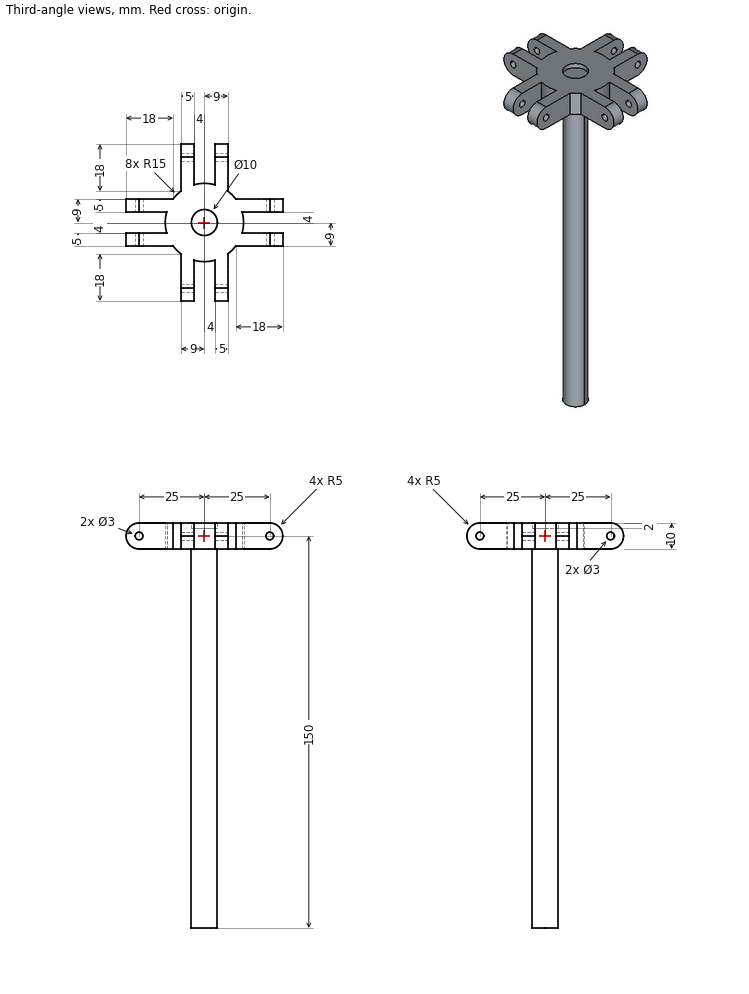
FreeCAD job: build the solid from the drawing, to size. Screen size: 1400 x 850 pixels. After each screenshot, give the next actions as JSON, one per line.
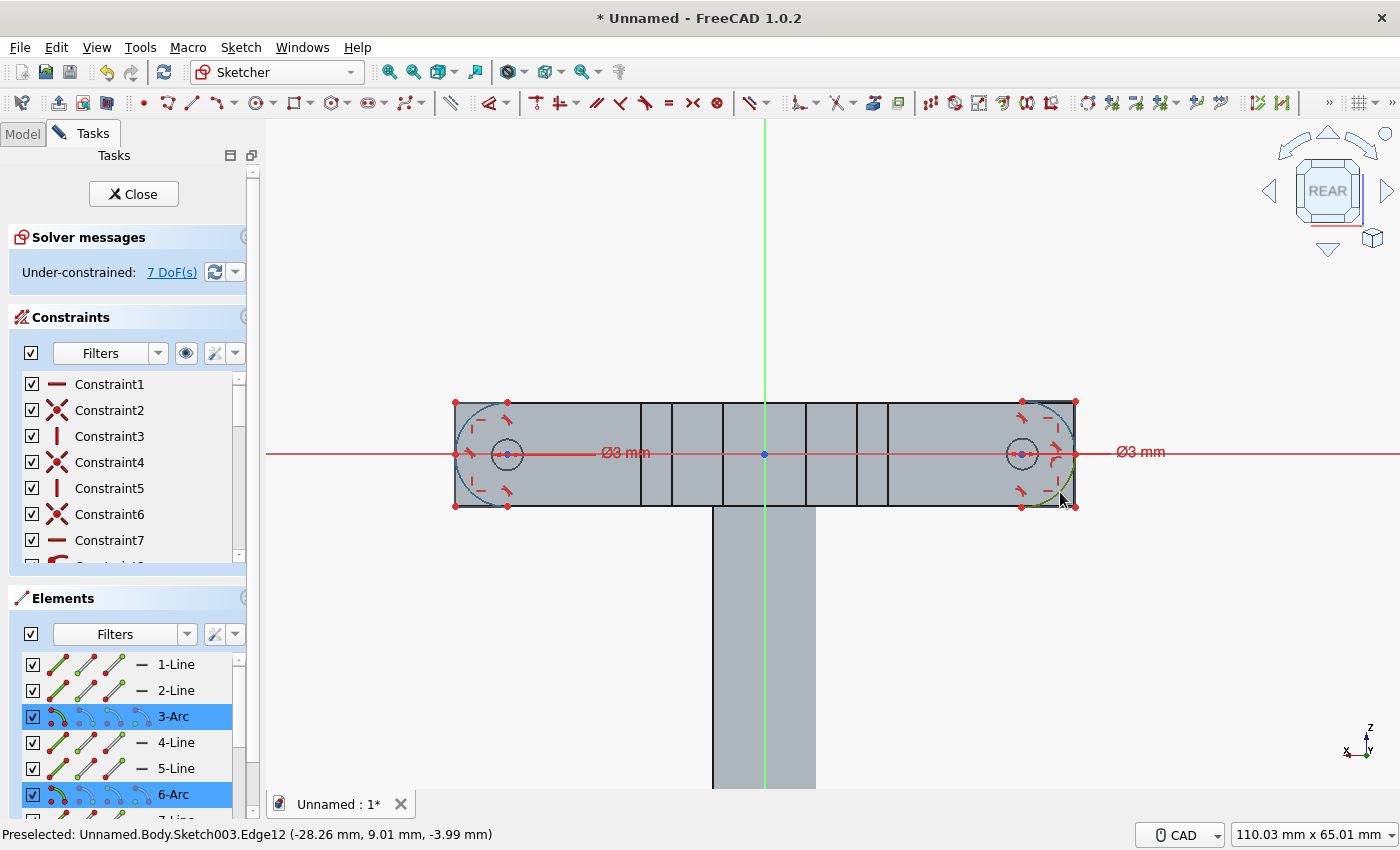
{"action": "key", "text": "e"}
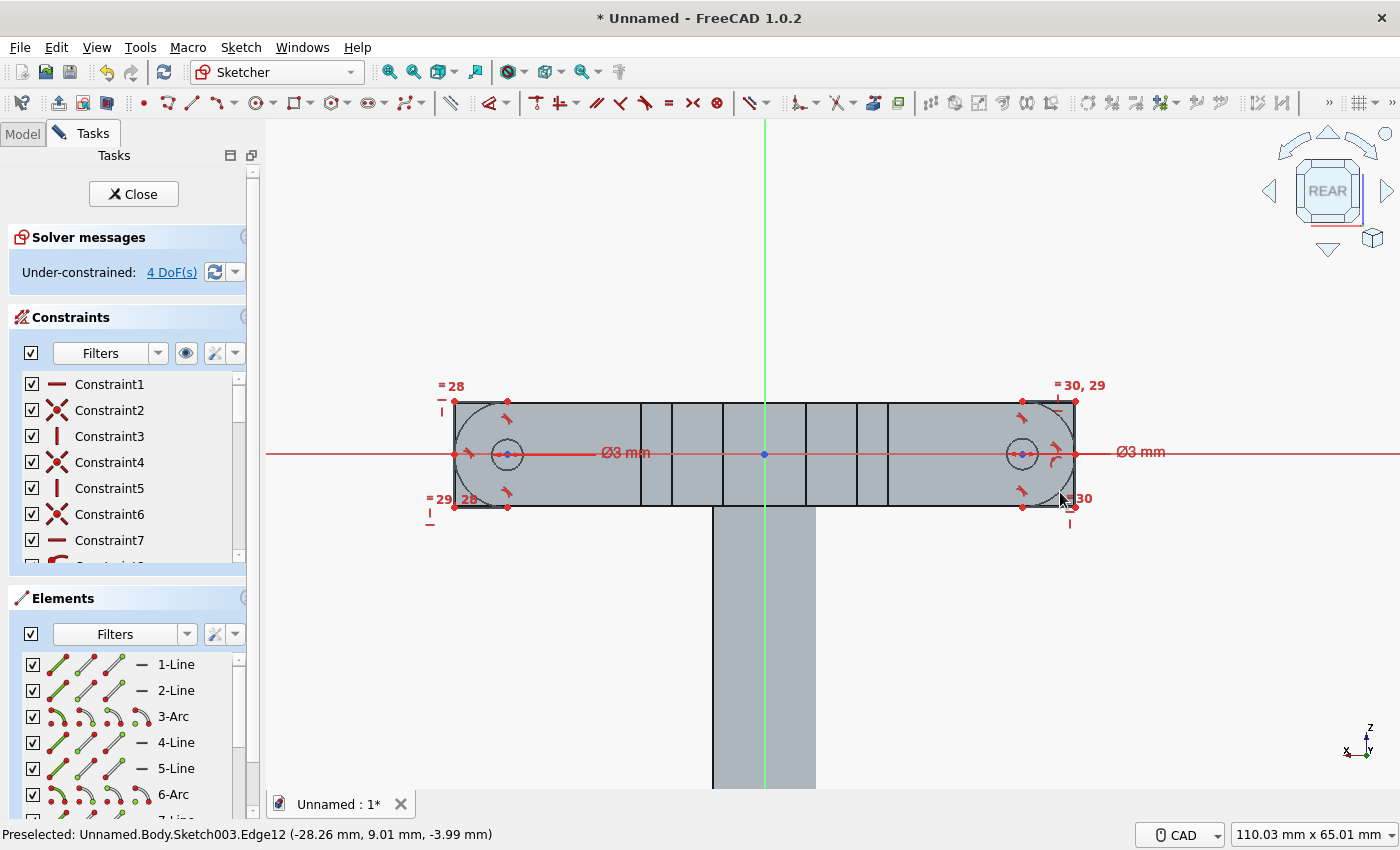
{"action": "left_click", "coordinate": [507, 455]}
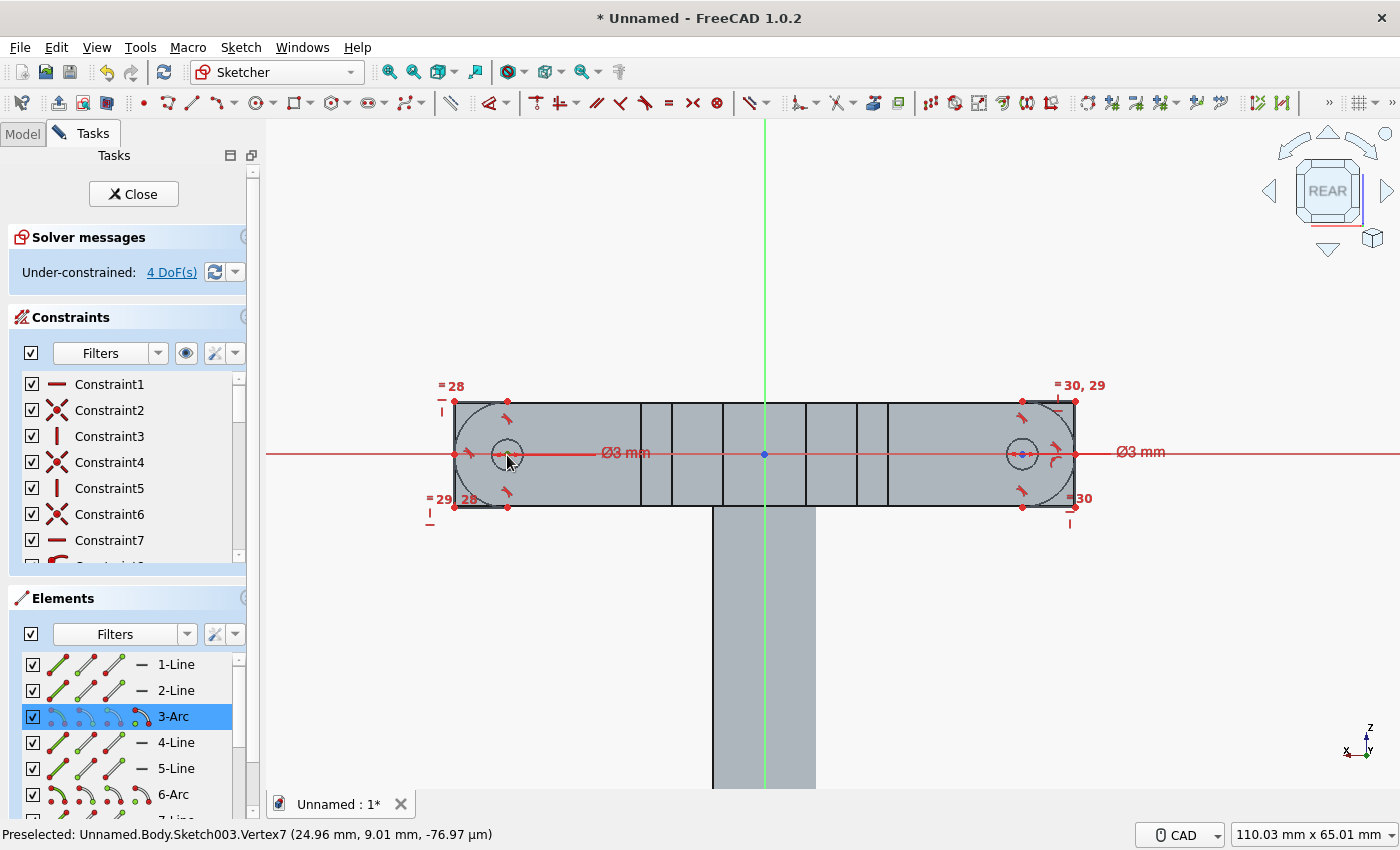
{"action": "left_click", "coordinate": [361, 454]}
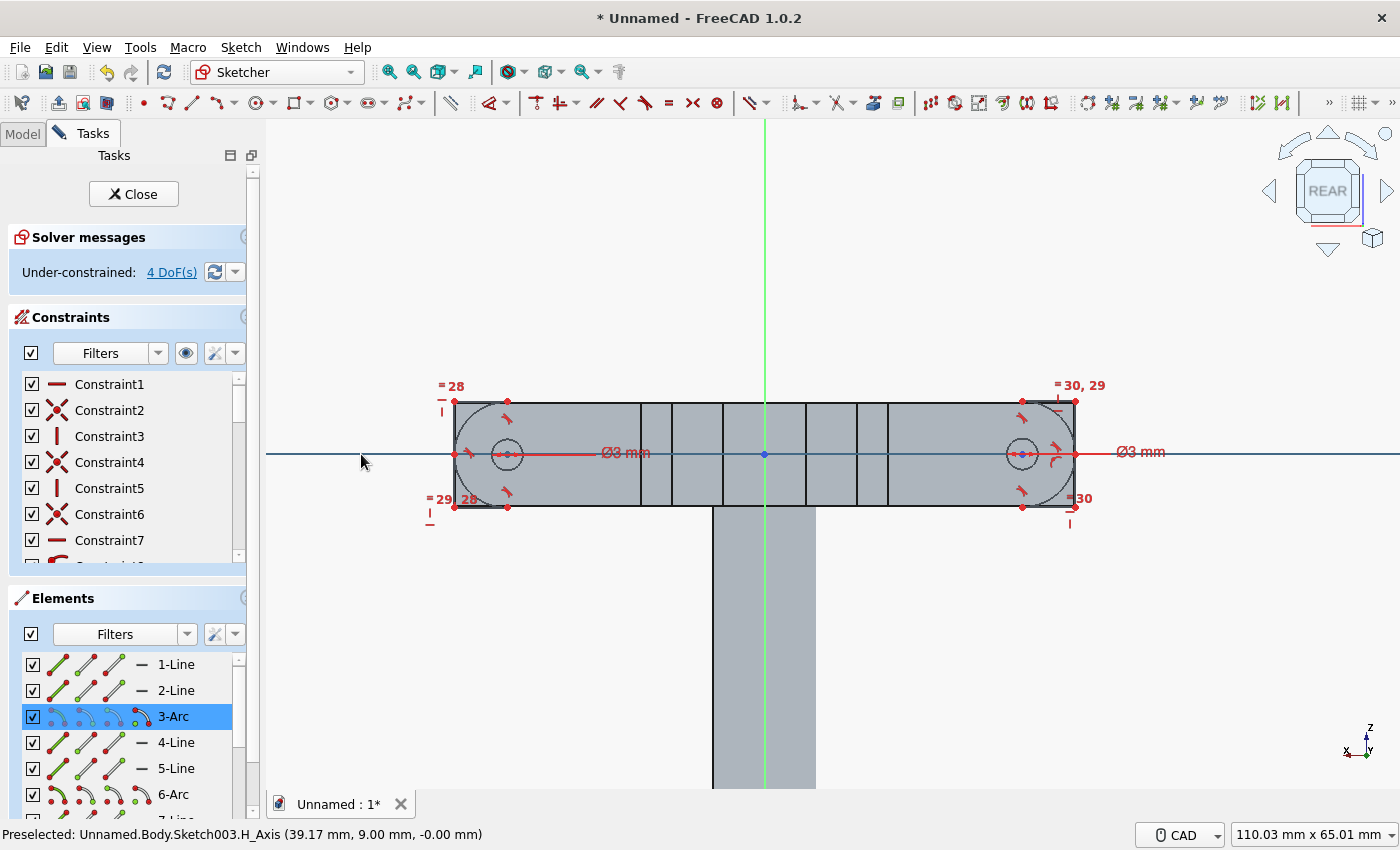
{"action": "key", "text": "c"}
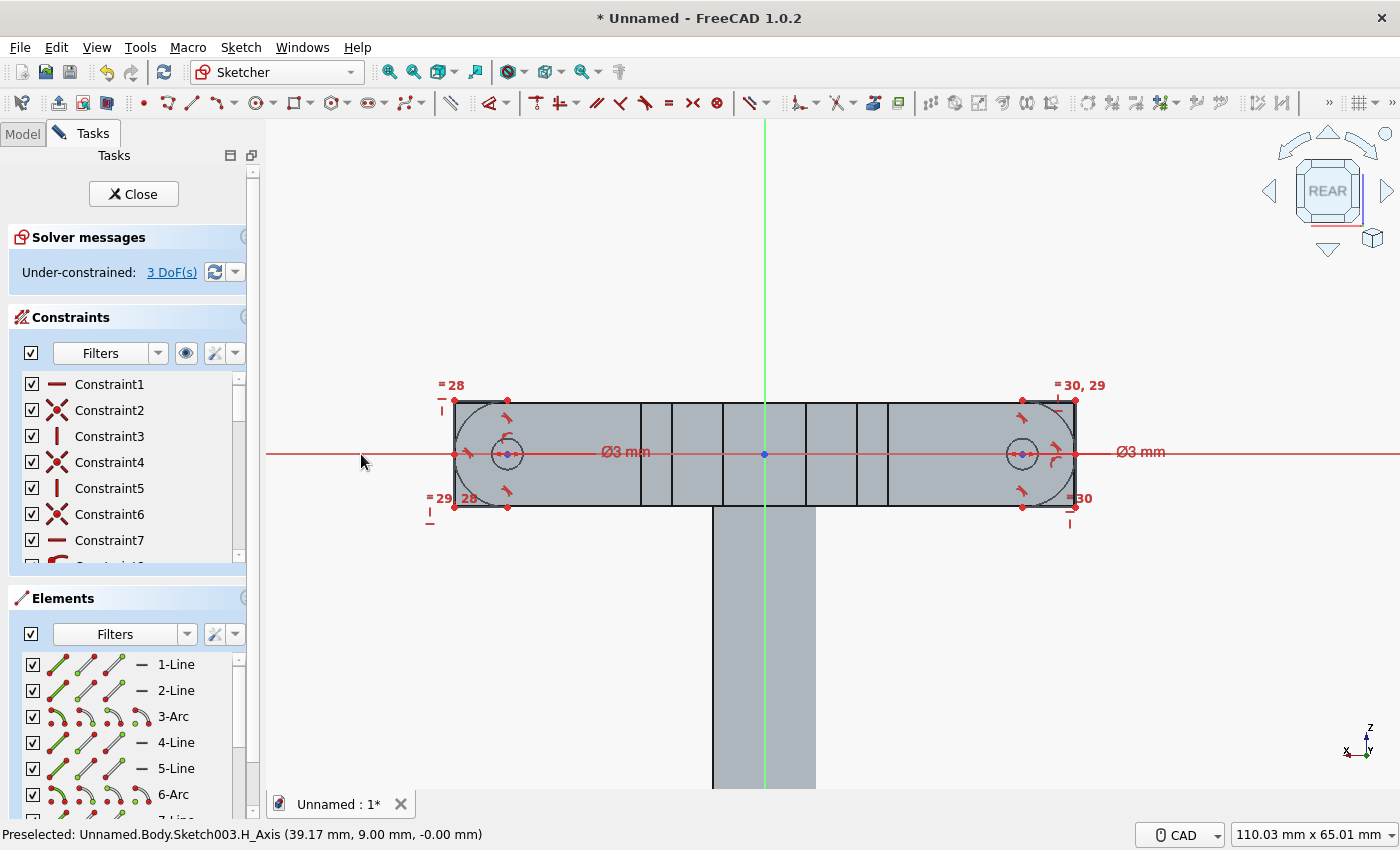
{"action": "key", "text": "d"}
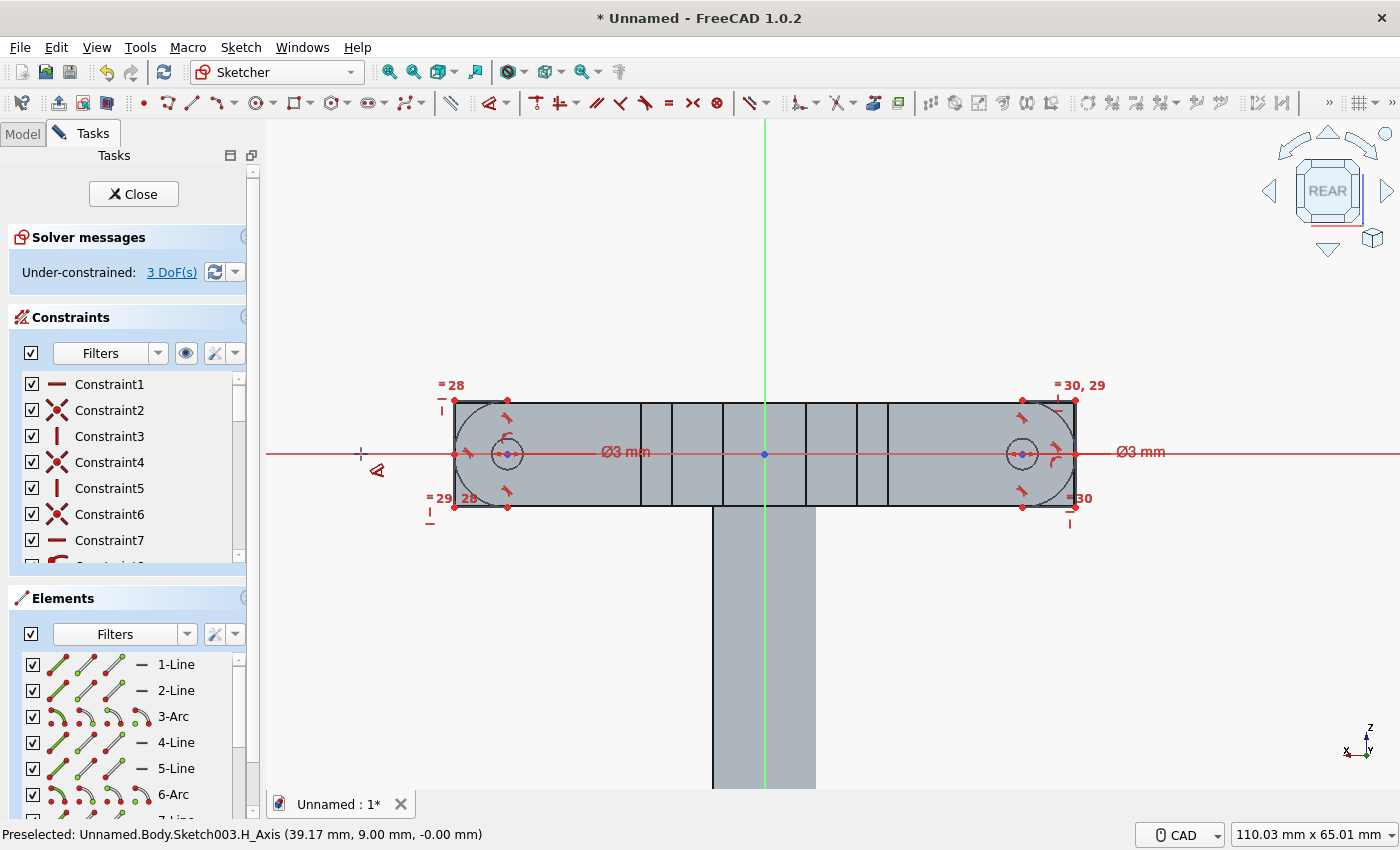
{"action": "left_click", "coordinate": [470, 416]}
{"action": "left_click", "coordinate": [484, 372]}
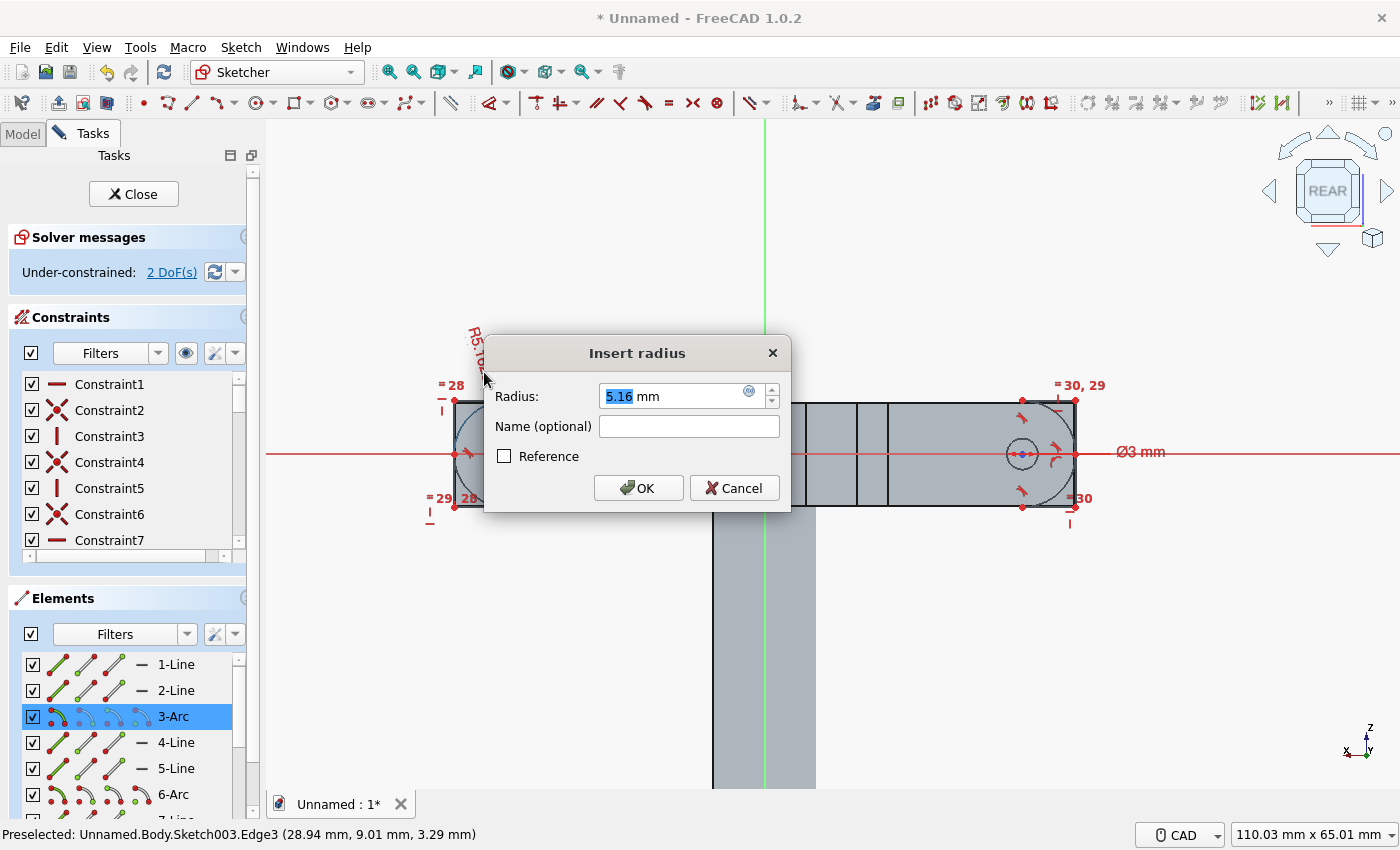
{"action": "type", "text": "5"}
{"action": "key", "text": "Return"}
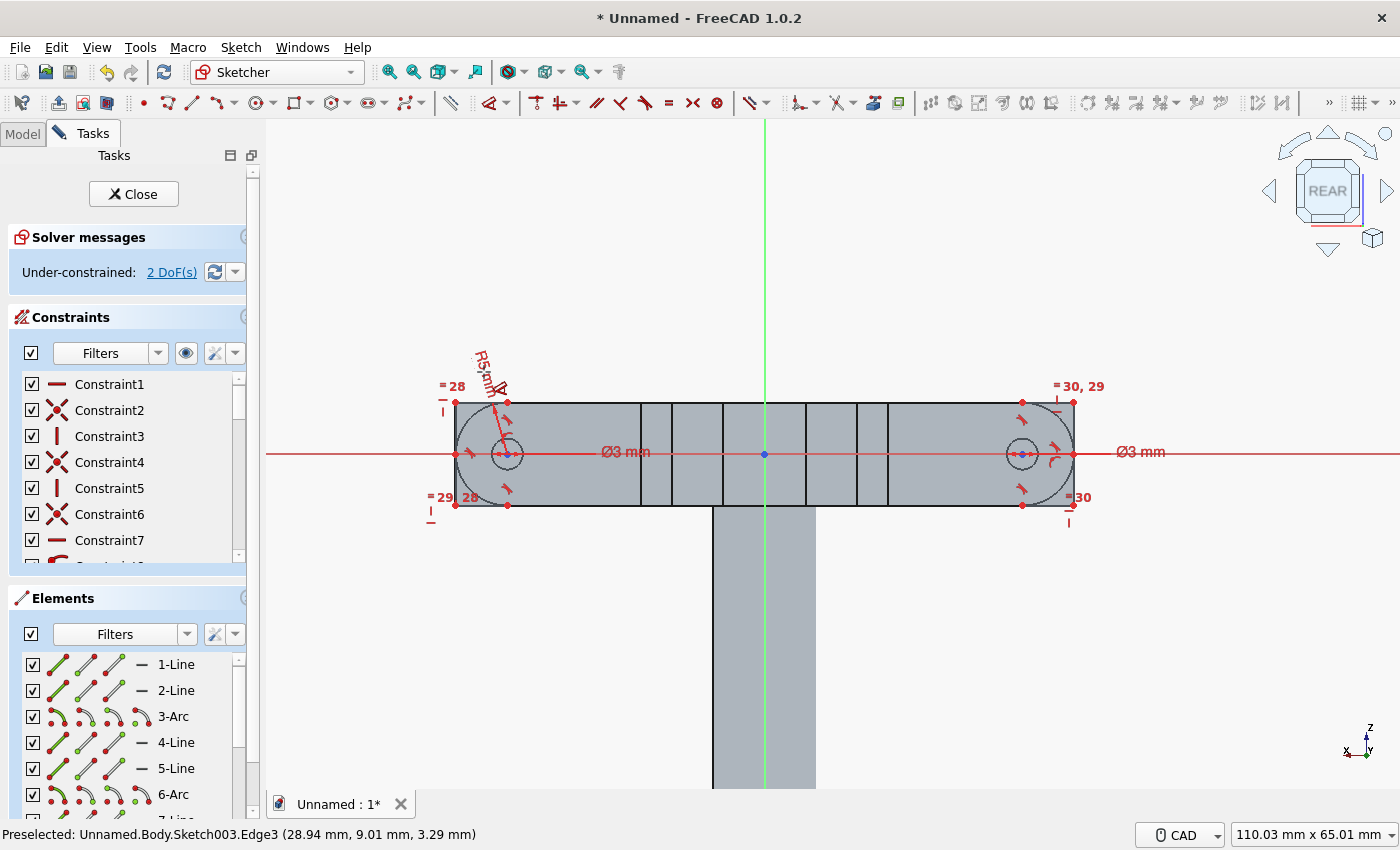
{"action": "left_click", "coordinate": [1022, 454]}
{"action": "left_click", "coordinate": [894, 488]}